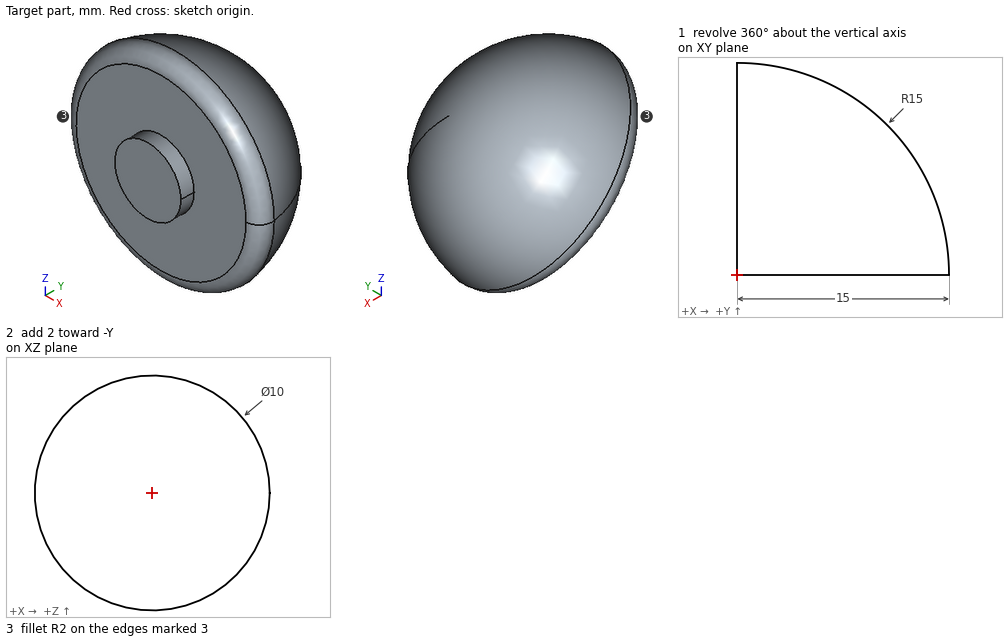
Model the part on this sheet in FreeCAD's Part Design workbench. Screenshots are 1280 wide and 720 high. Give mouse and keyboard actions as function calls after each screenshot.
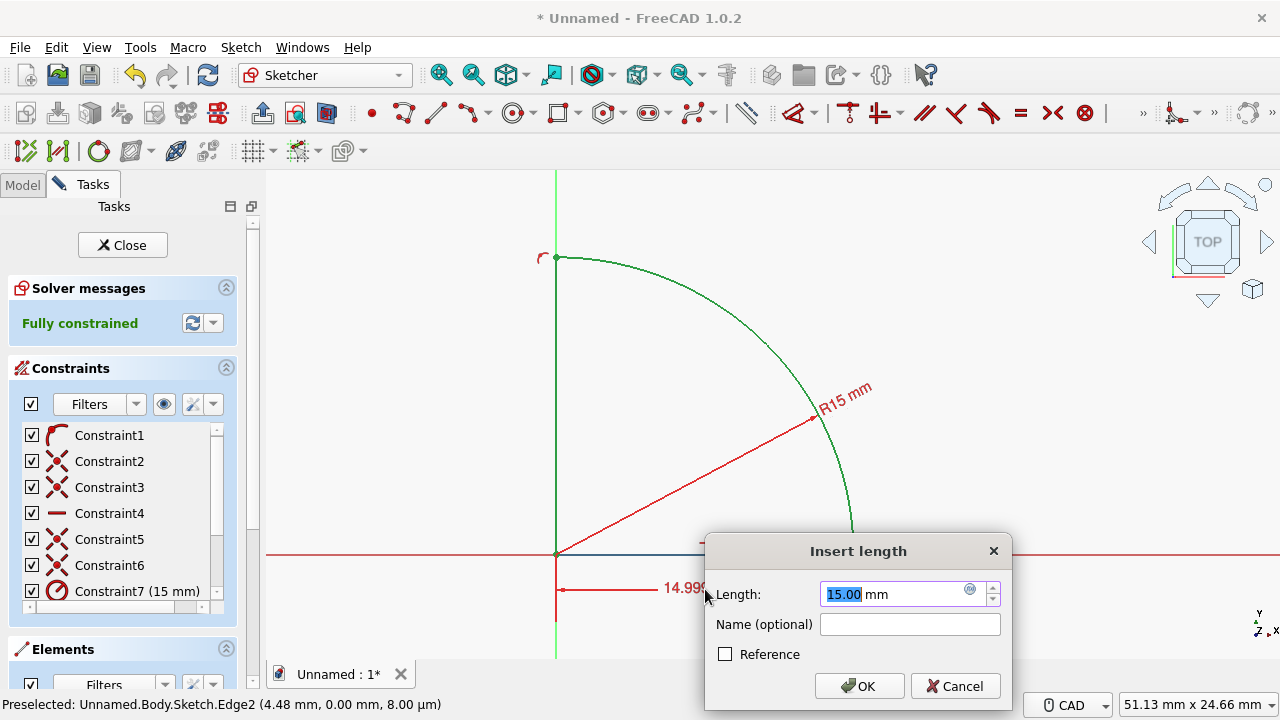
text(15)
key(Return)
key(Escape)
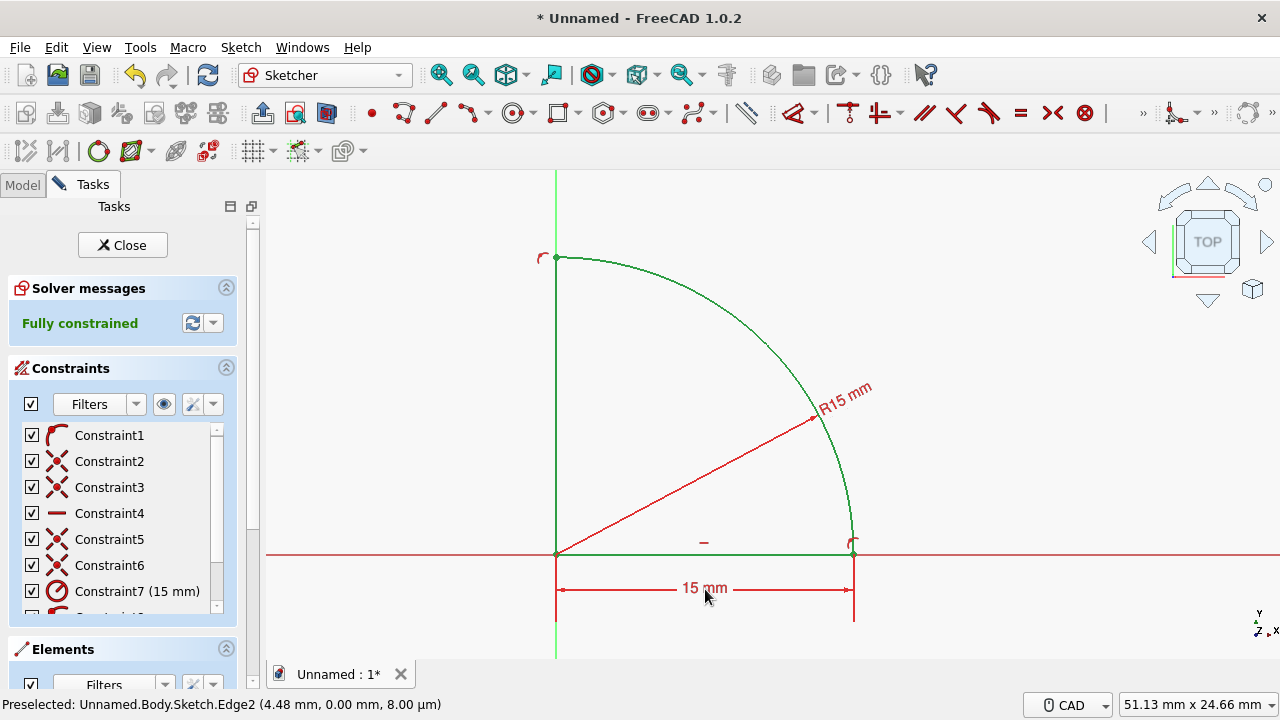
click(123, 245)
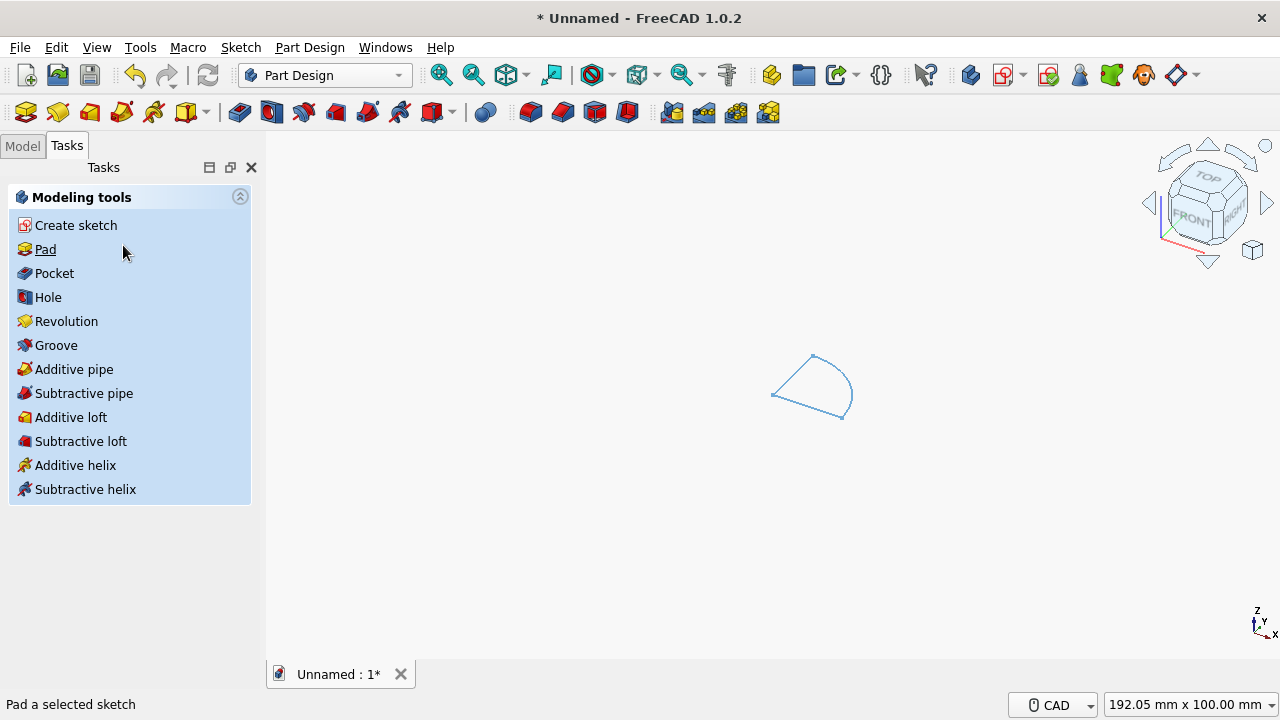
click(58, 112)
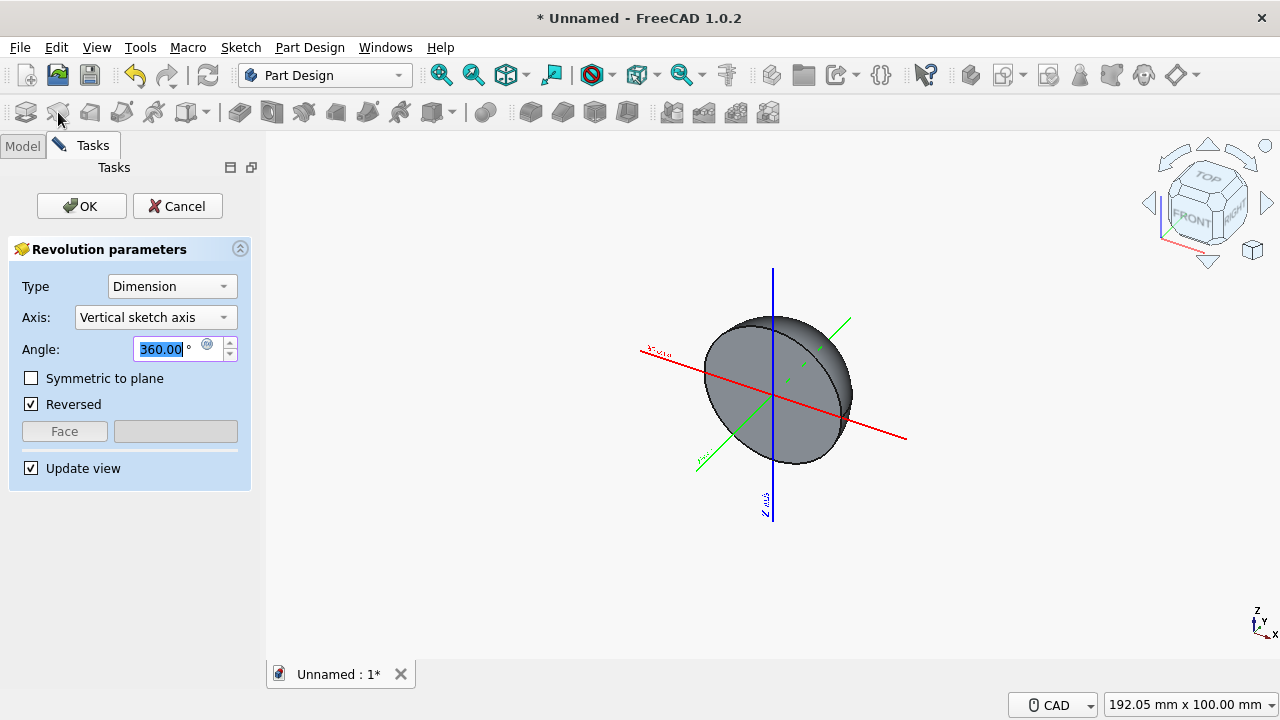
click(82, 206)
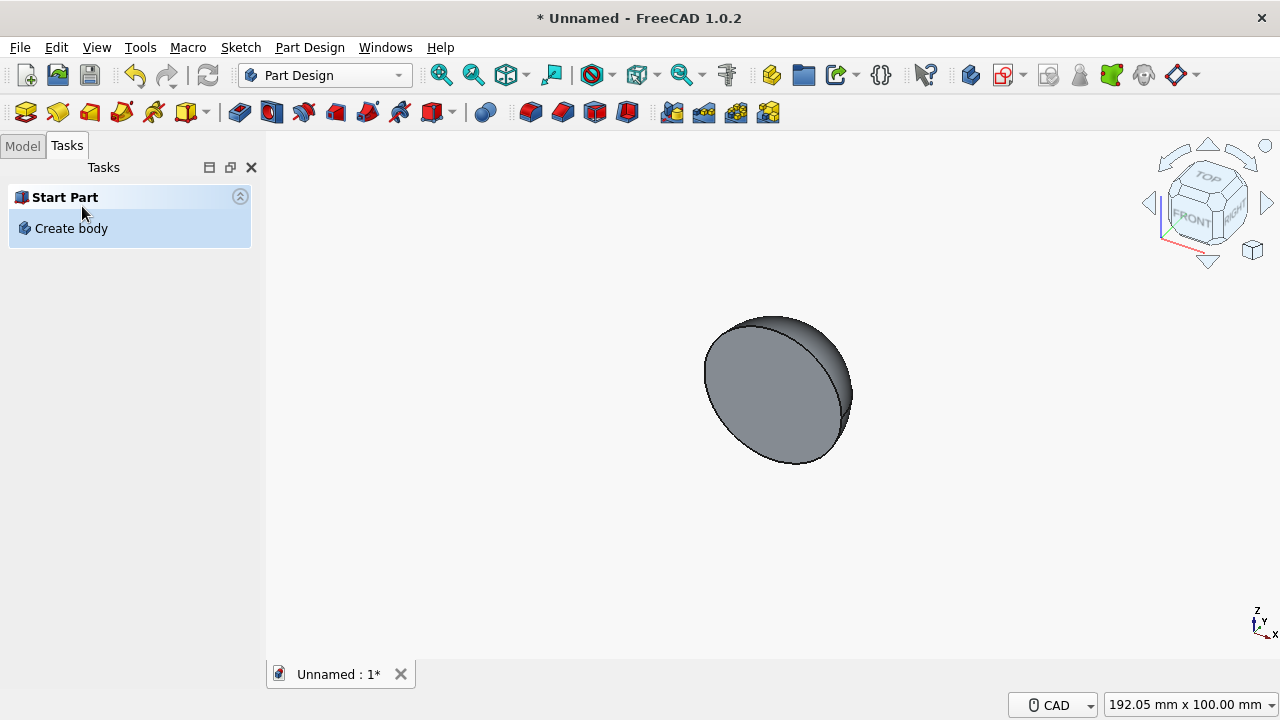
click(442, 76)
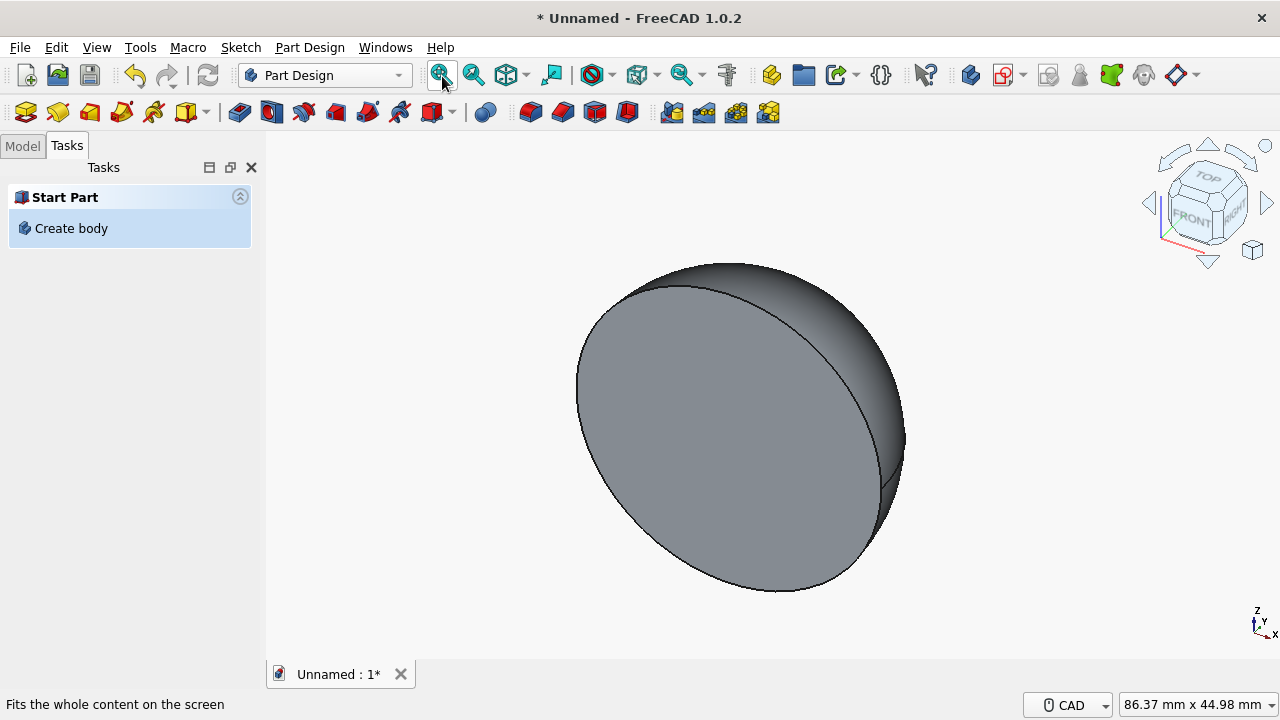
click(1004, 76)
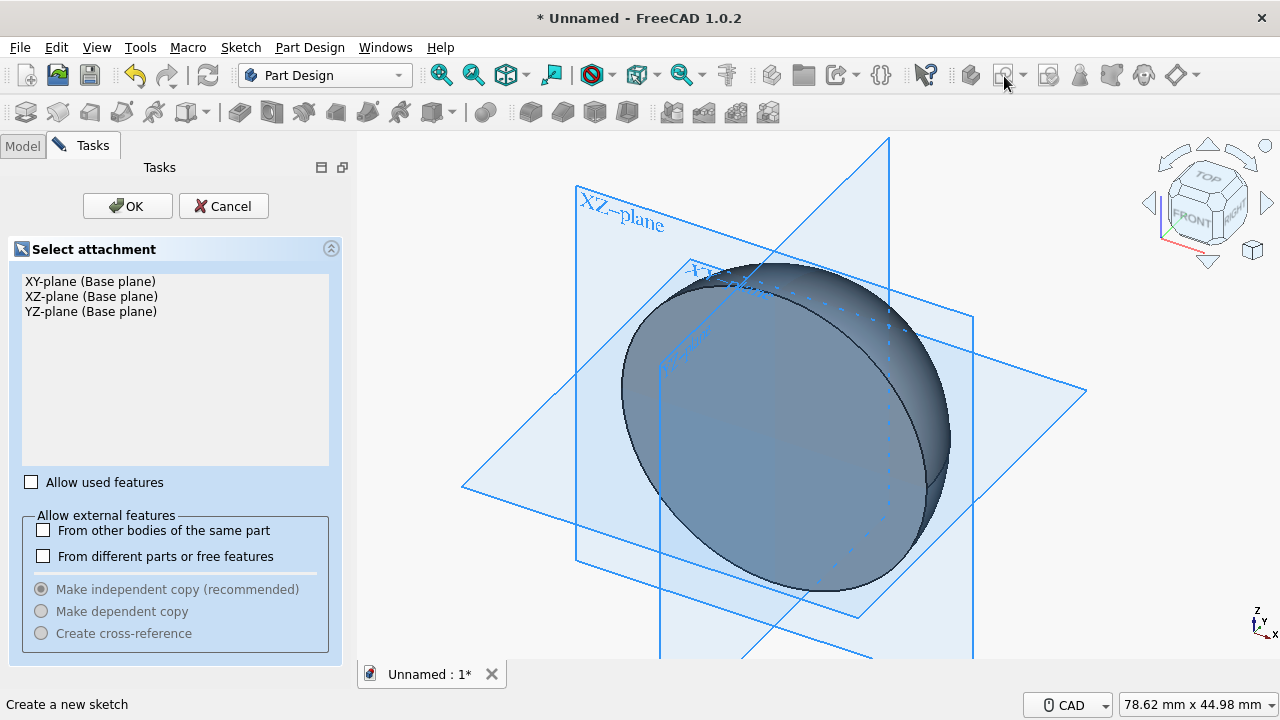
click(82, 296)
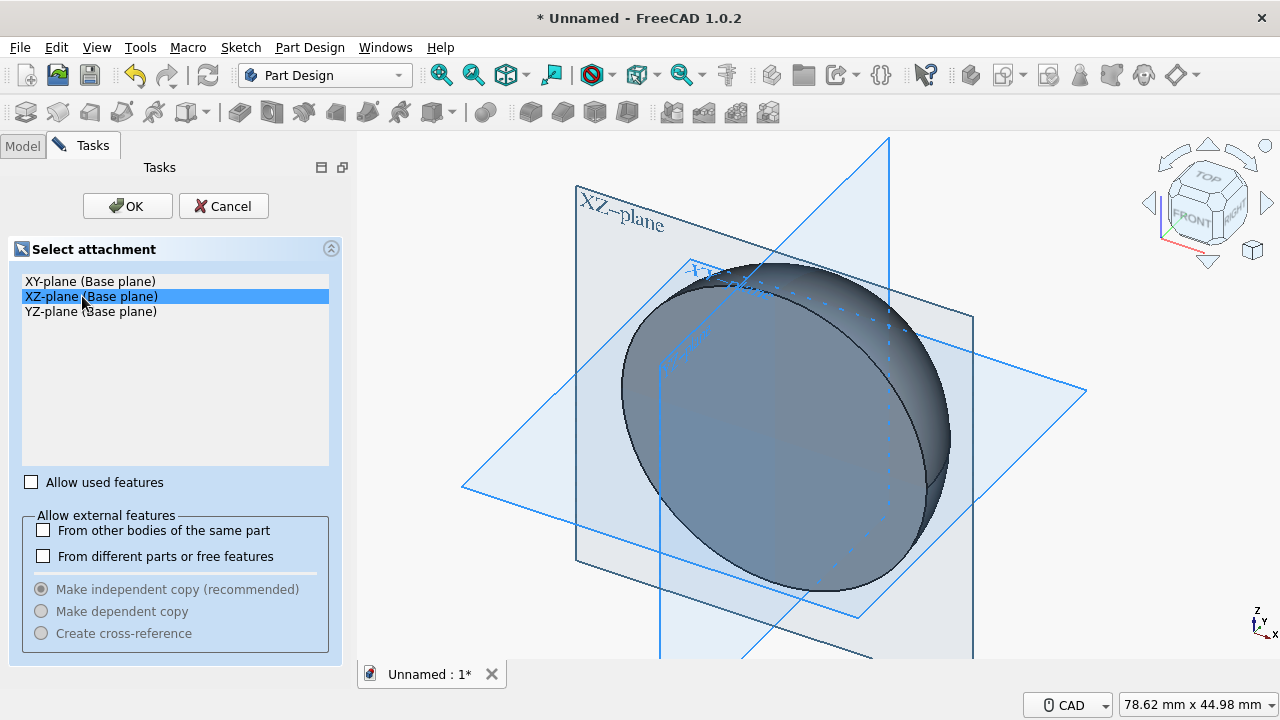
click(128, 206)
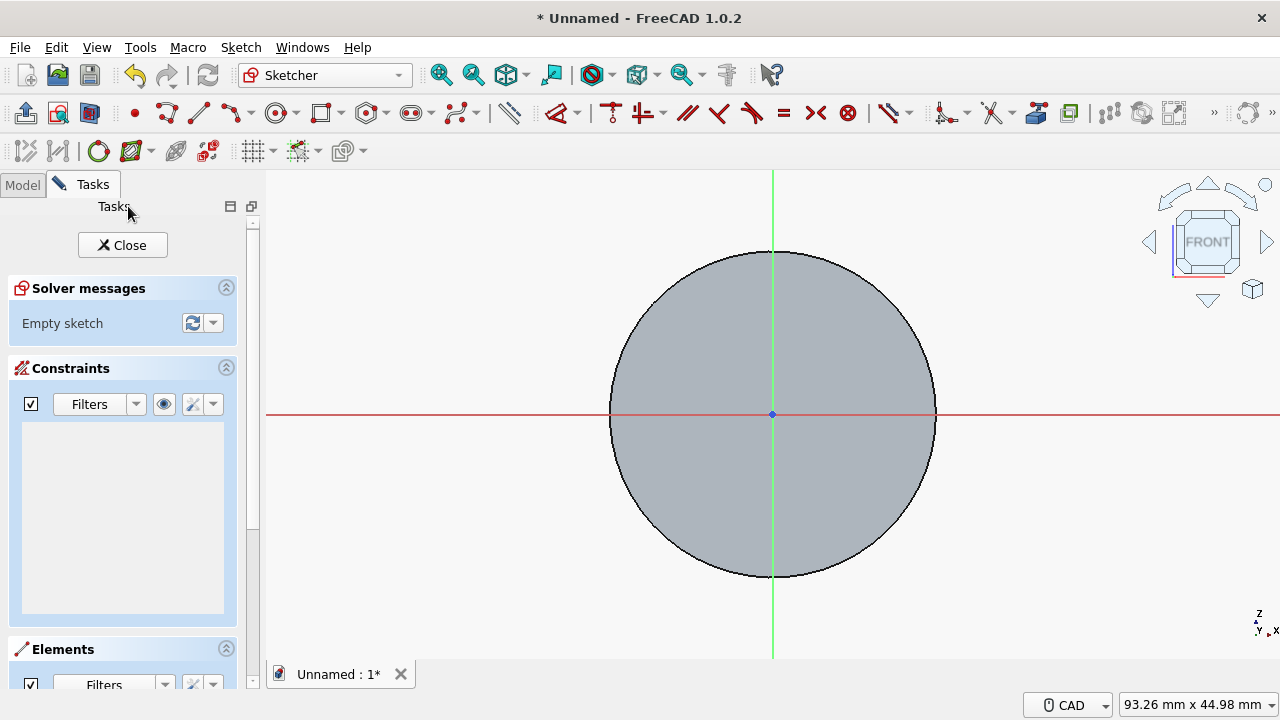
scroll(813, 415, up, 5)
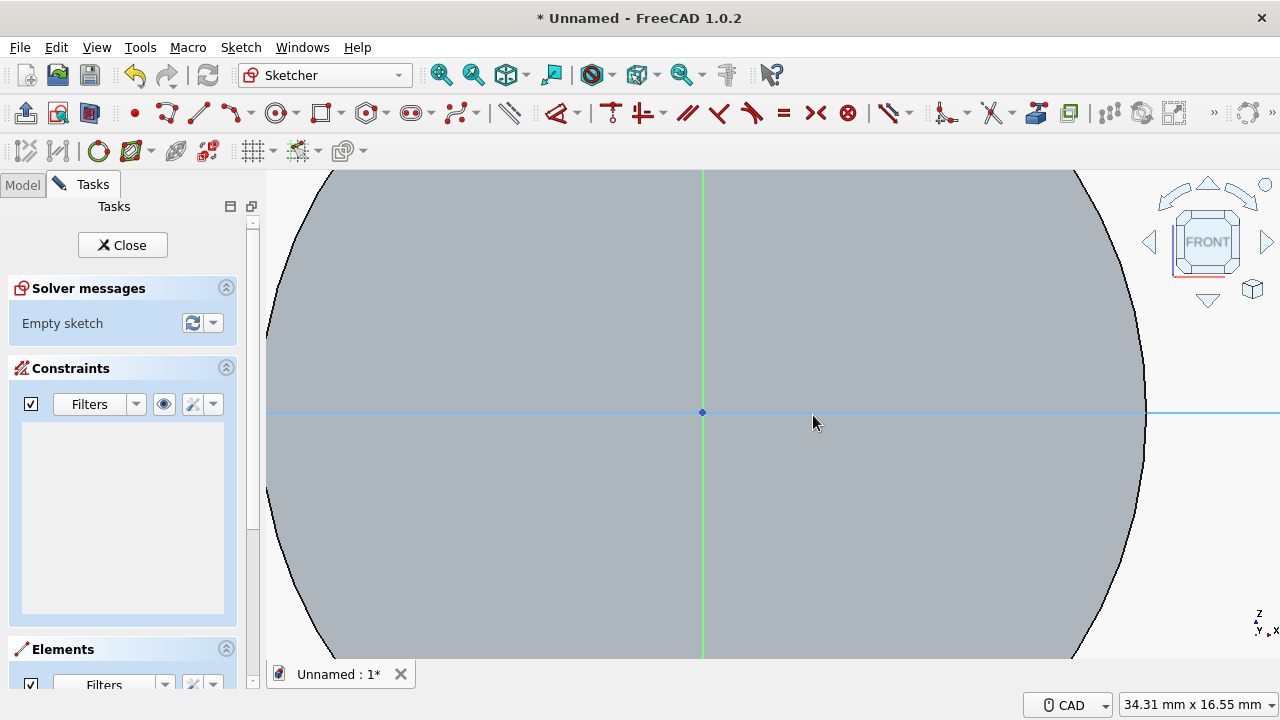
key(g)
key(c)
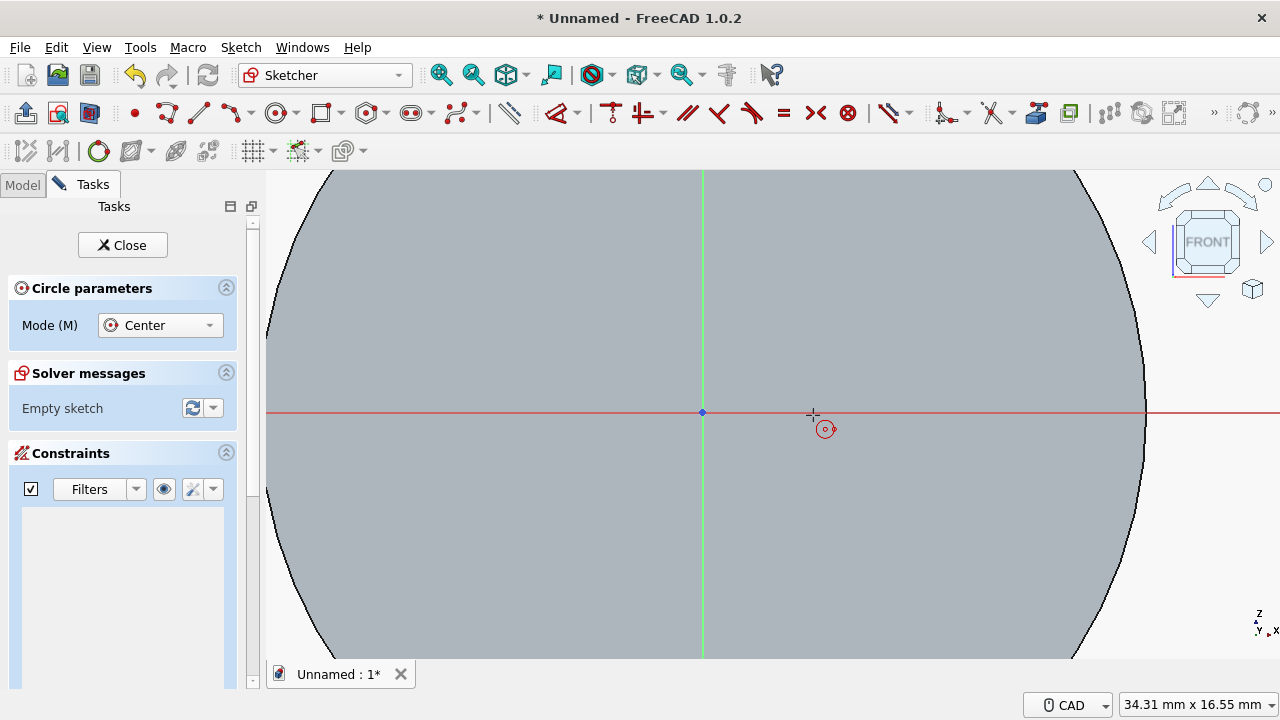
click(703, 413)
move(807, 308)